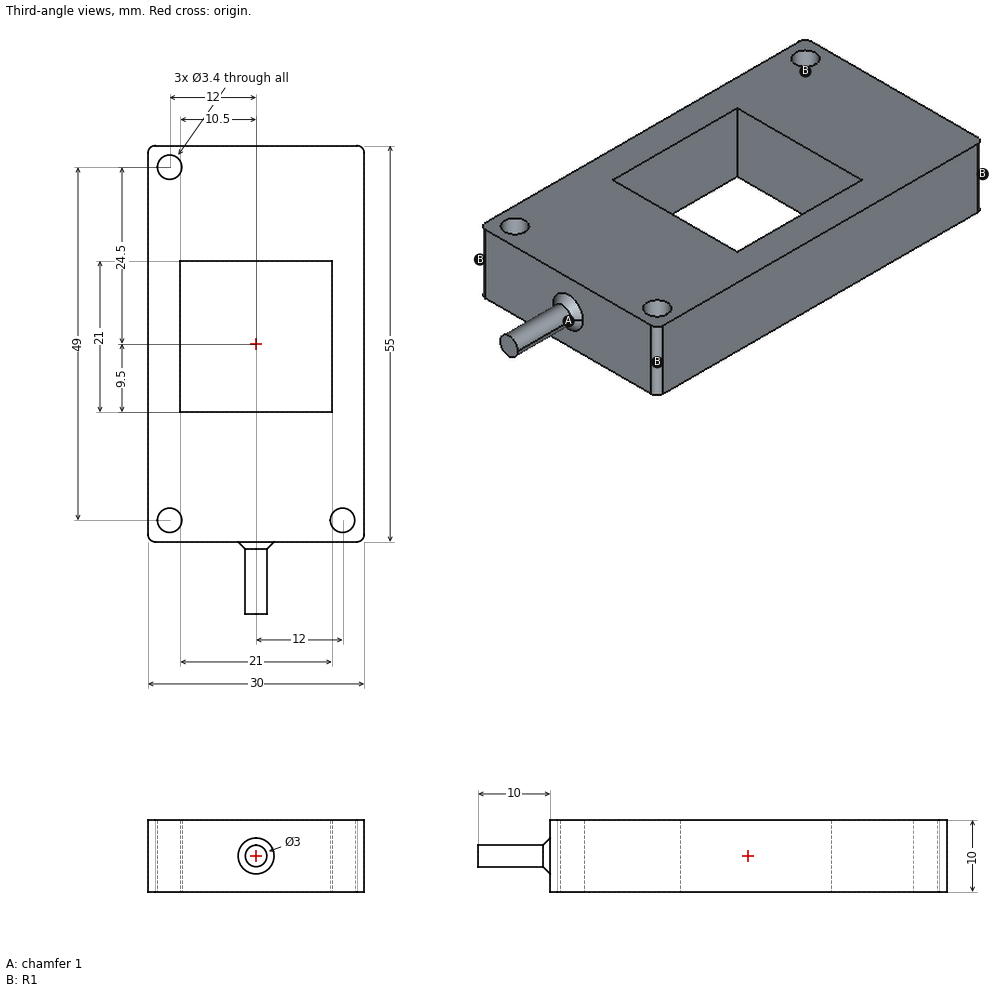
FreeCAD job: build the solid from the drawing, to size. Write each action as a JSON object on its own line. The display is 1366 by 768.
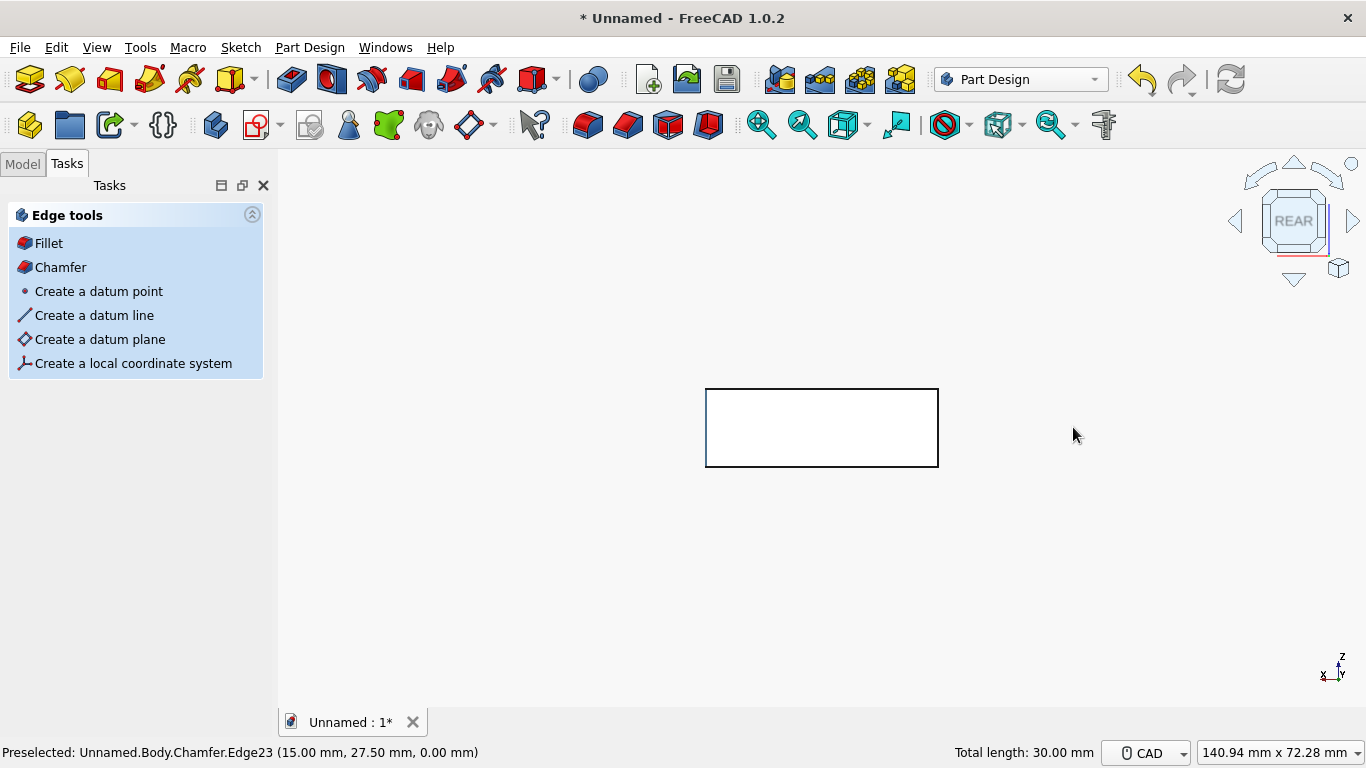
{"action": "left_click", "coordinate": [762, 126]}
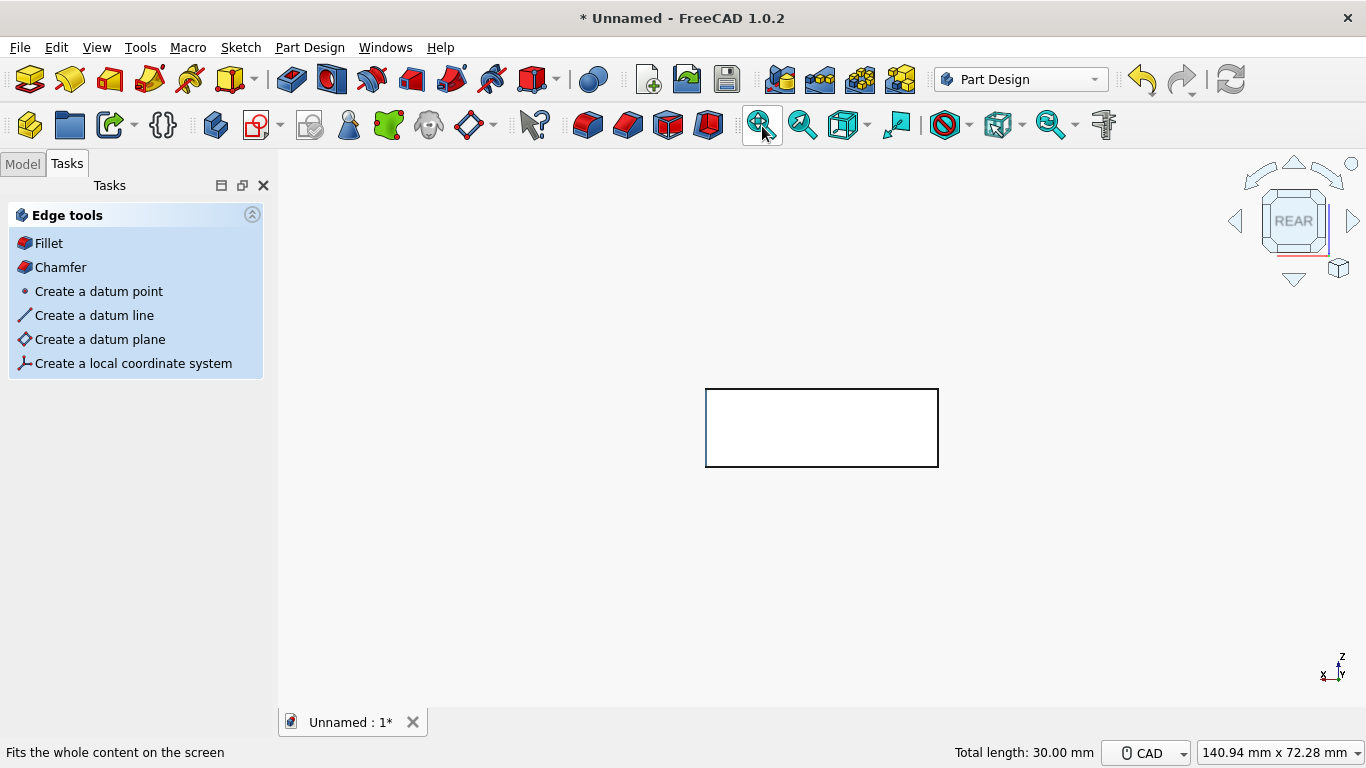
{"action": "left_click", "coordinate": [938, 427], "text": "ctrl"}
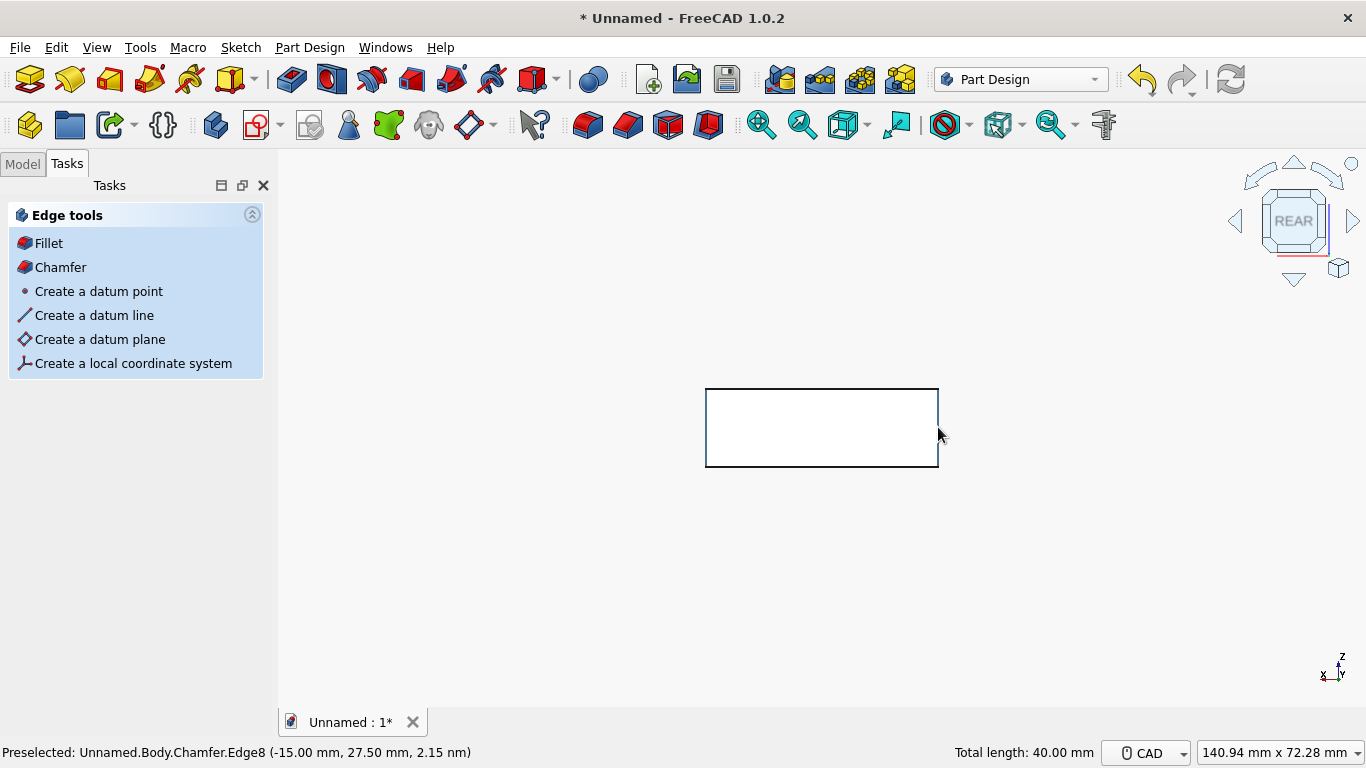
{"action": "left_click", "coordinate": [588, 126]}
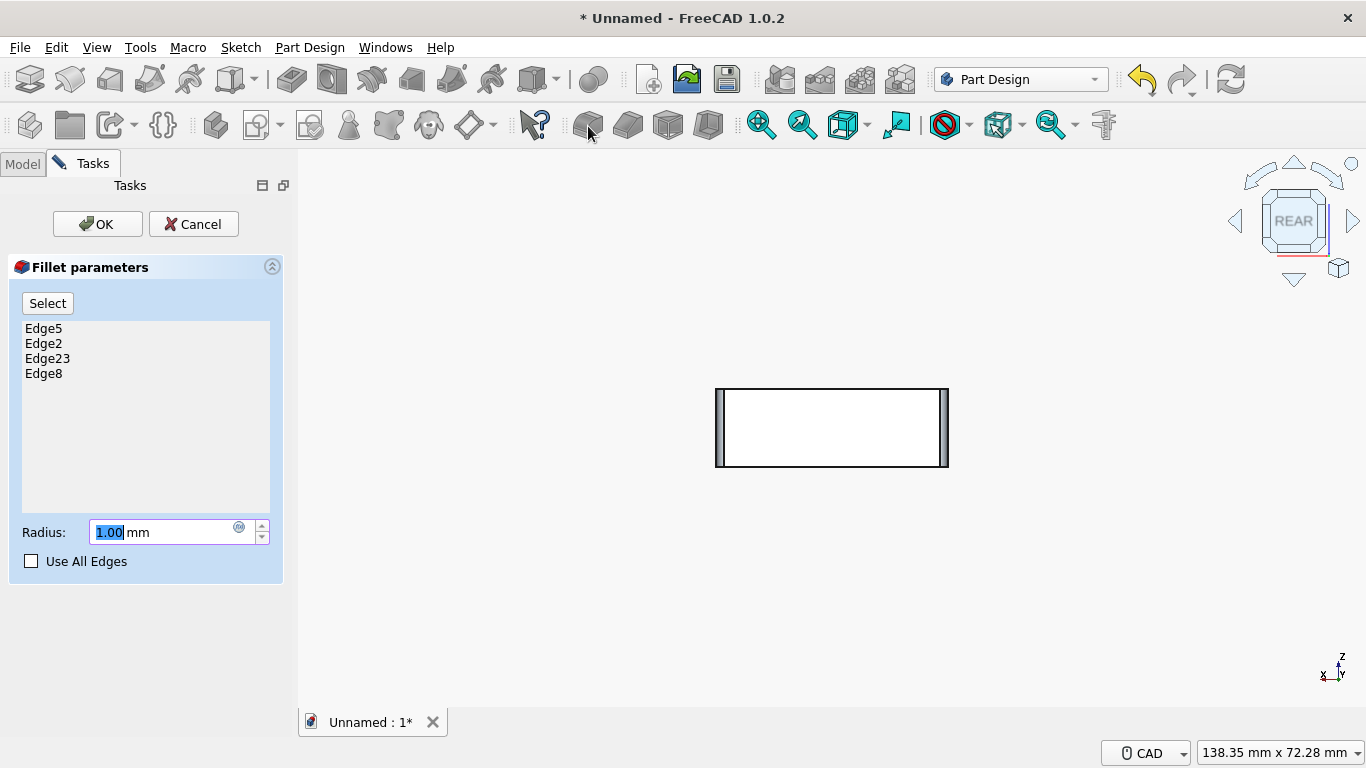
{"action": "type", "text": "1"}
{"action": "key", "text": "Tab"}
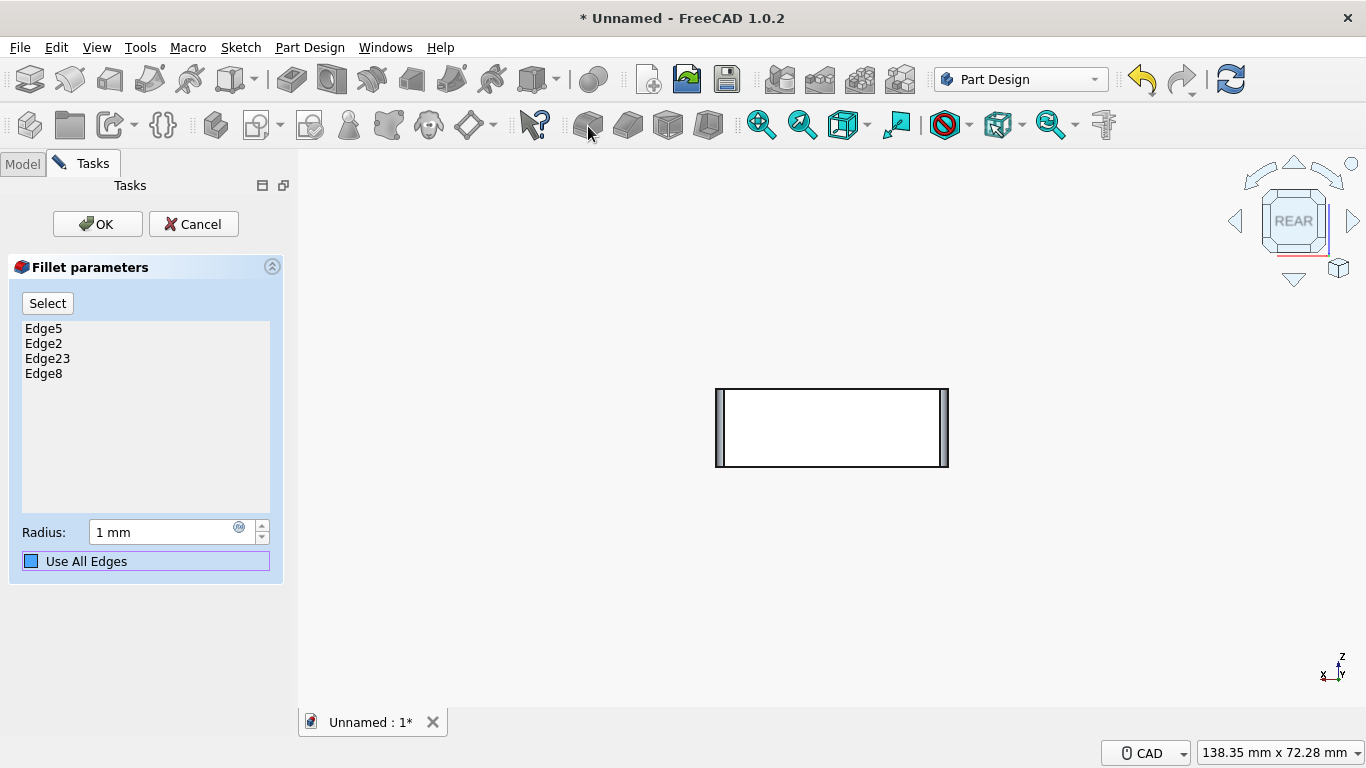
{"action": "left_click", "coordinate": [98, 224]}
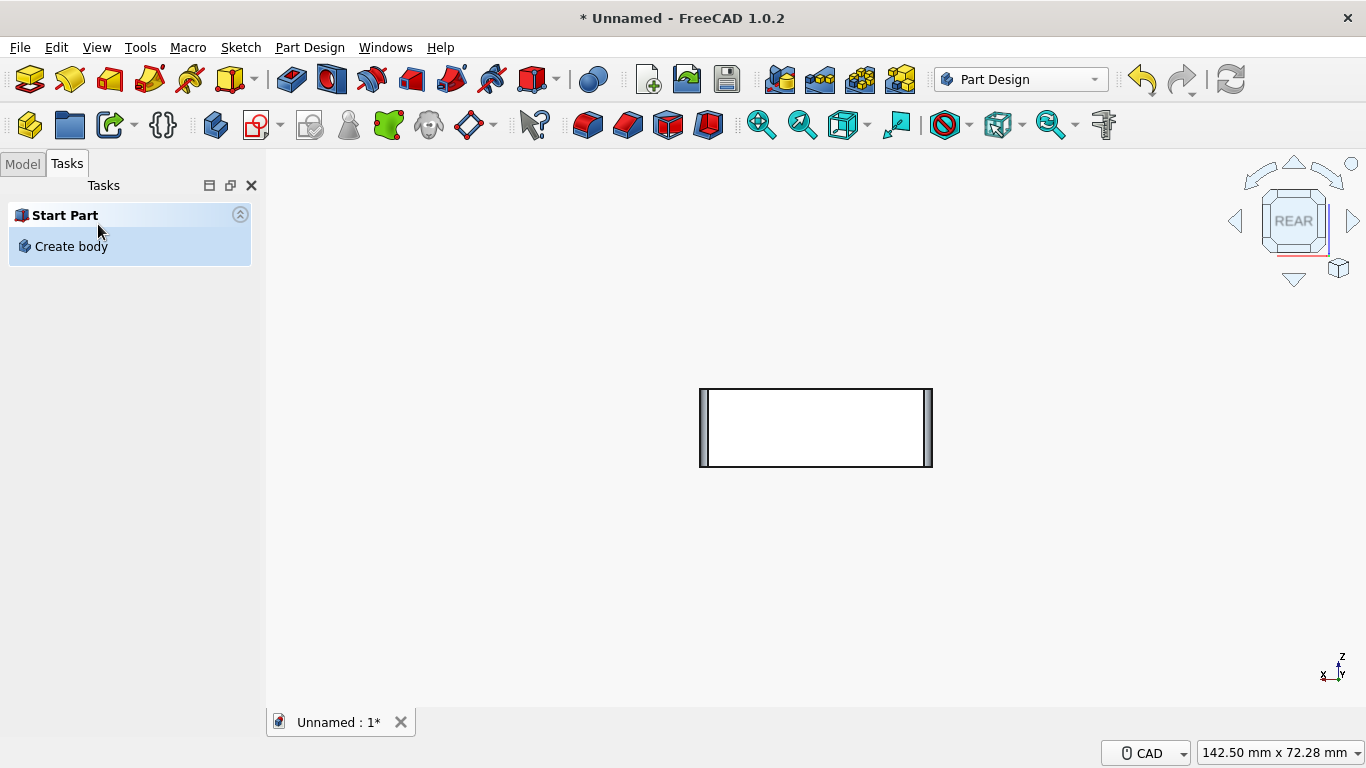
{"action": "key", "text": "v f"}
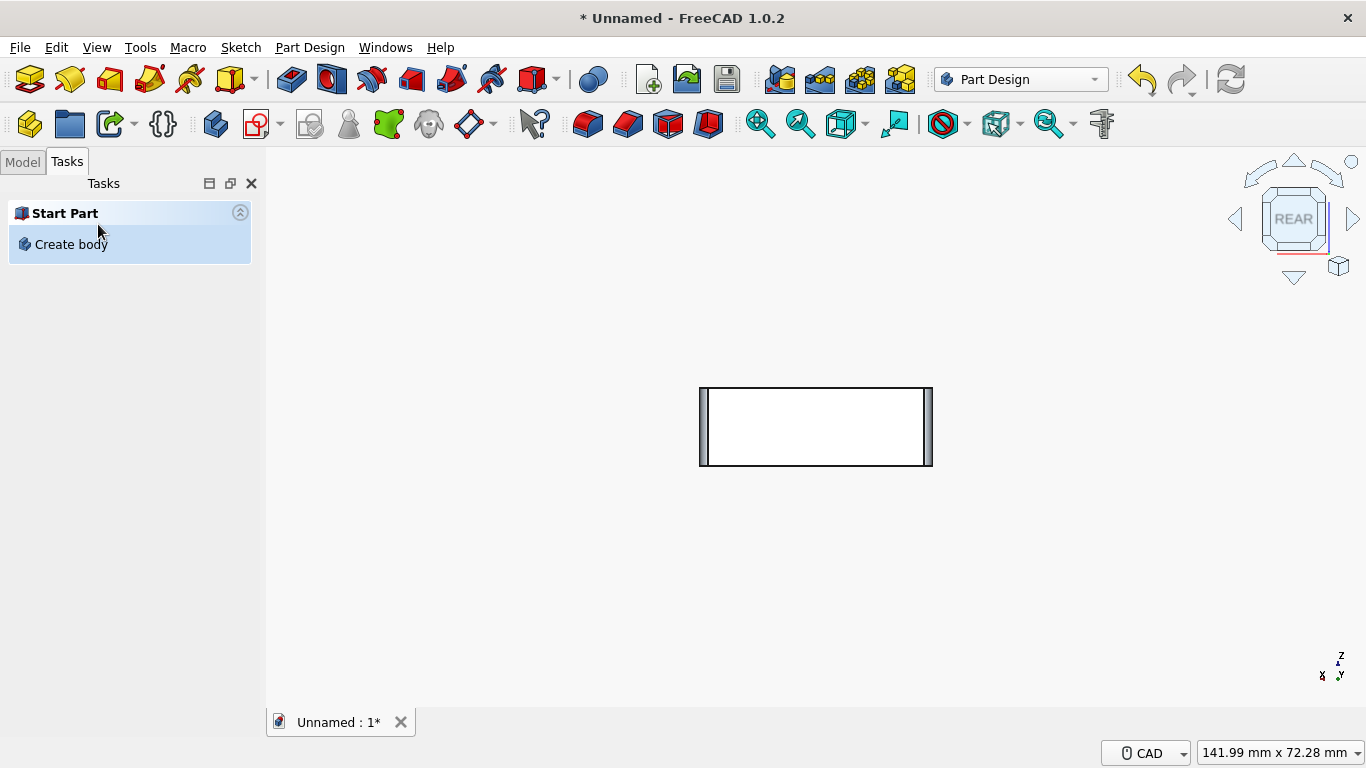
{"action": "key", "text": "0"}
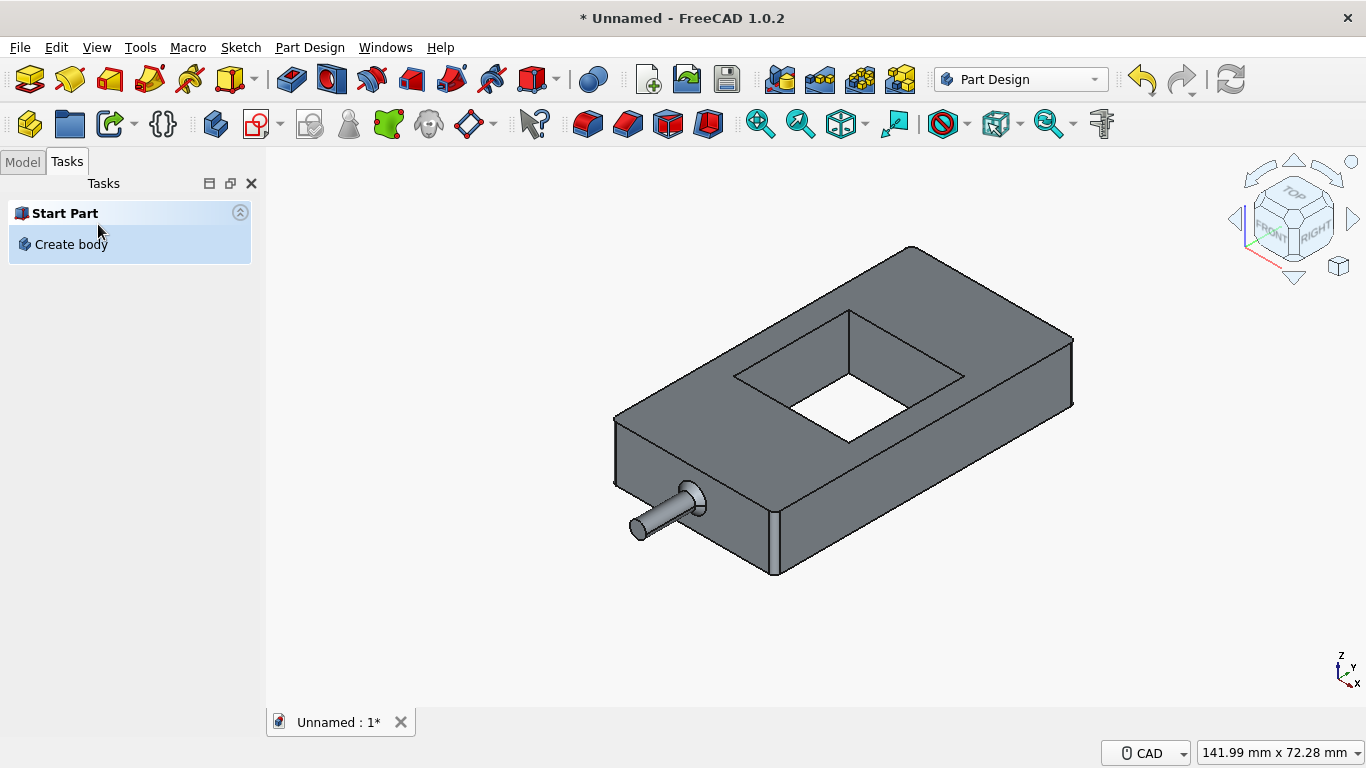
{"action": "left_click", "coordinate": [804, 455]}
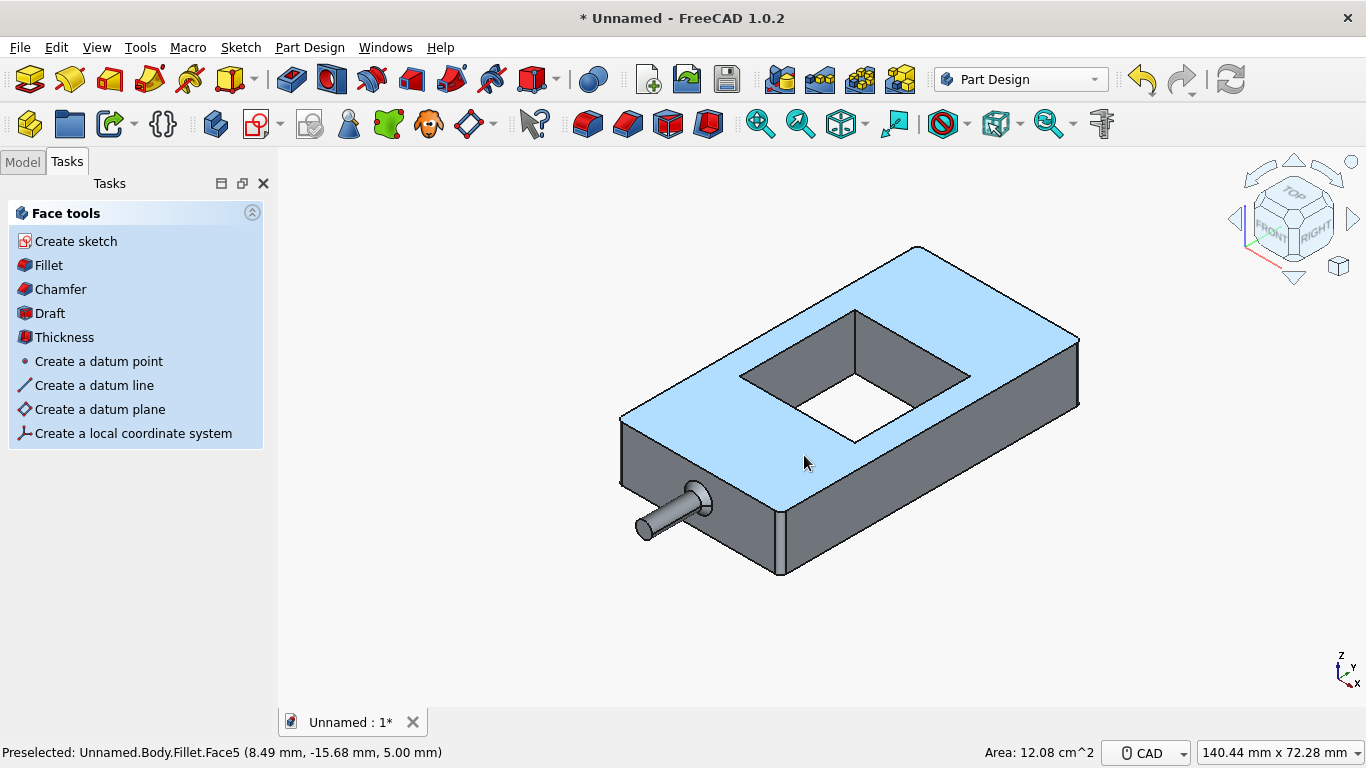
{"action": "left_click", "coordinate": [256, 124]}